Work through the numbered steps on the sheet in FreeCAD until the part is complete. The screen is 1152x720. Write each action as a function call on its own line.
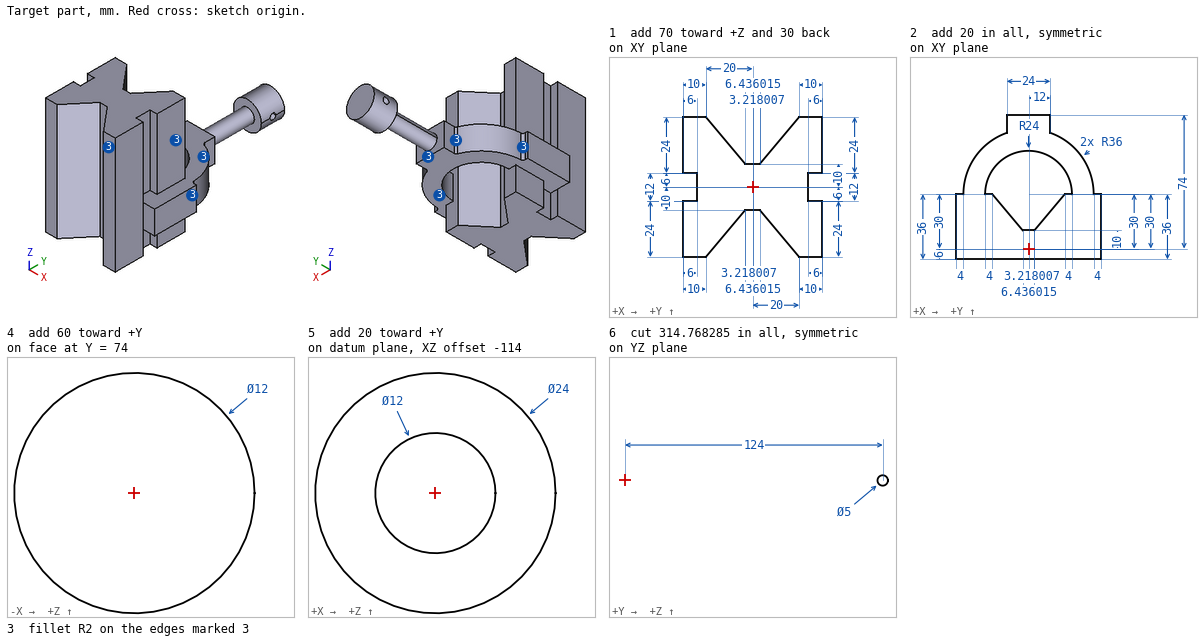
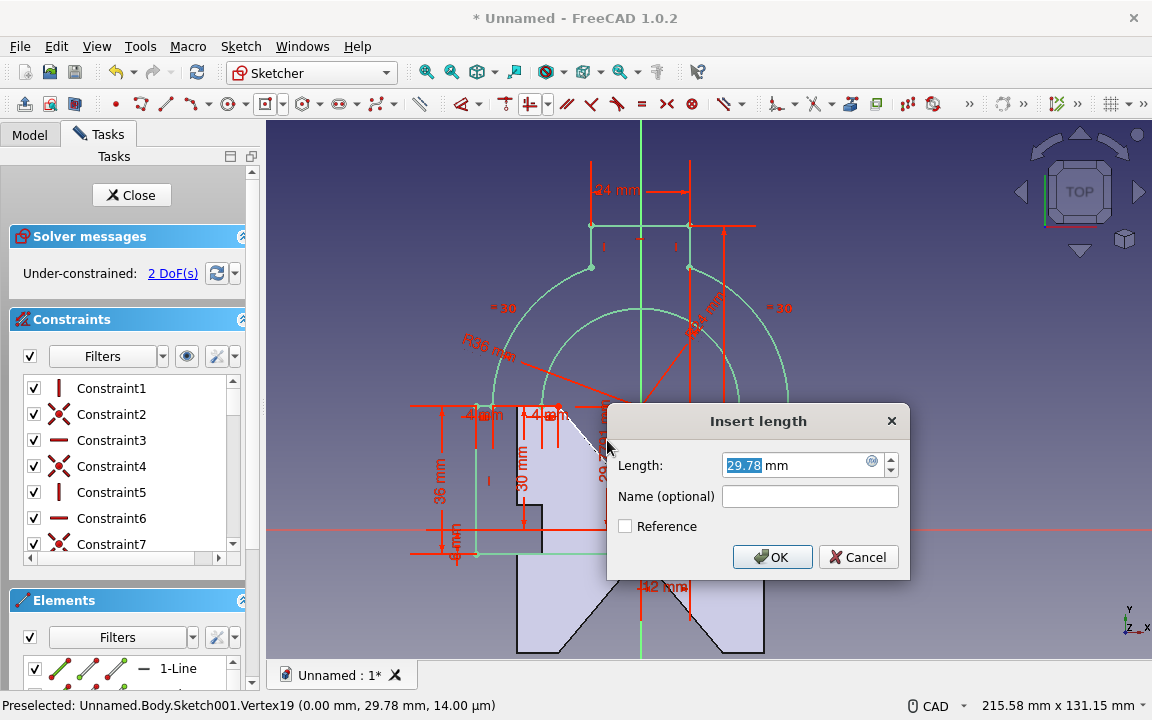
text(30)
key(Return)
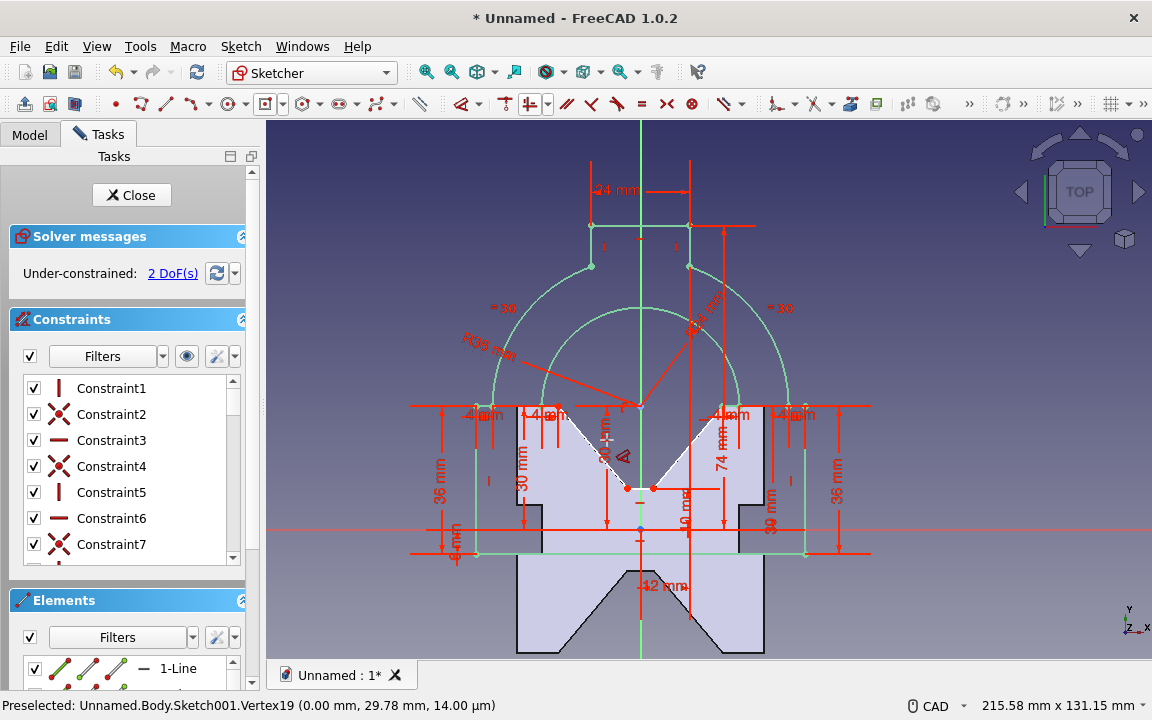
scroll(643, 489, up, 3)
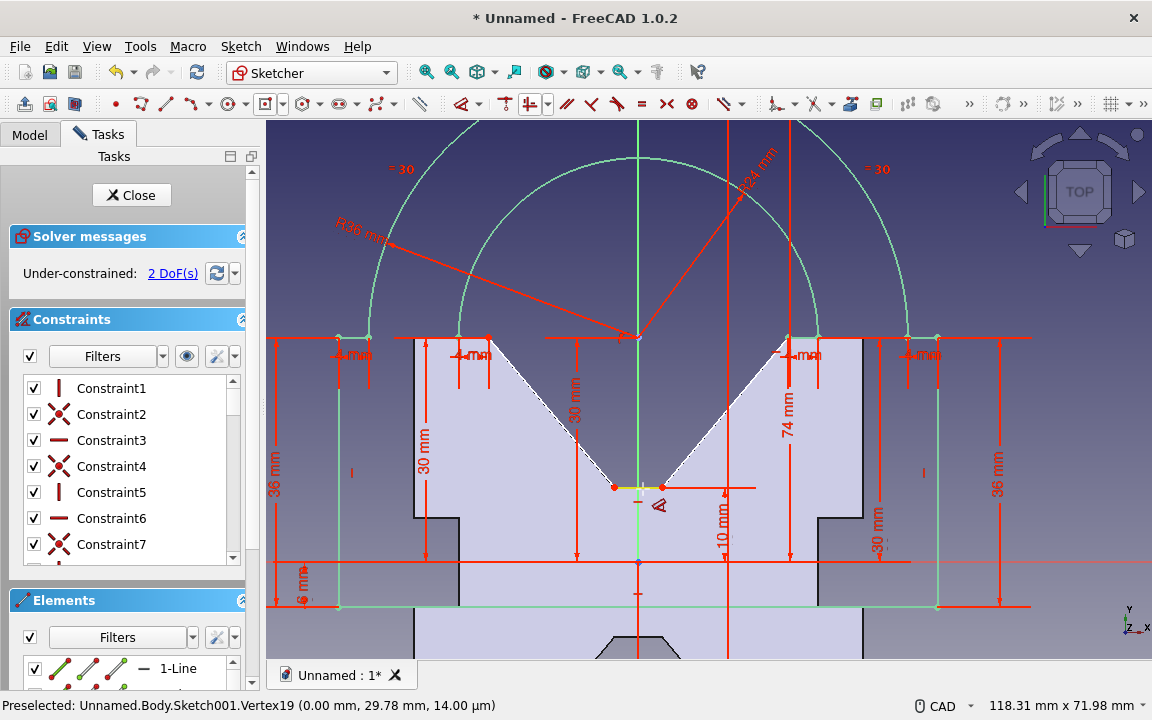
click(643, 488)
click(622, 522)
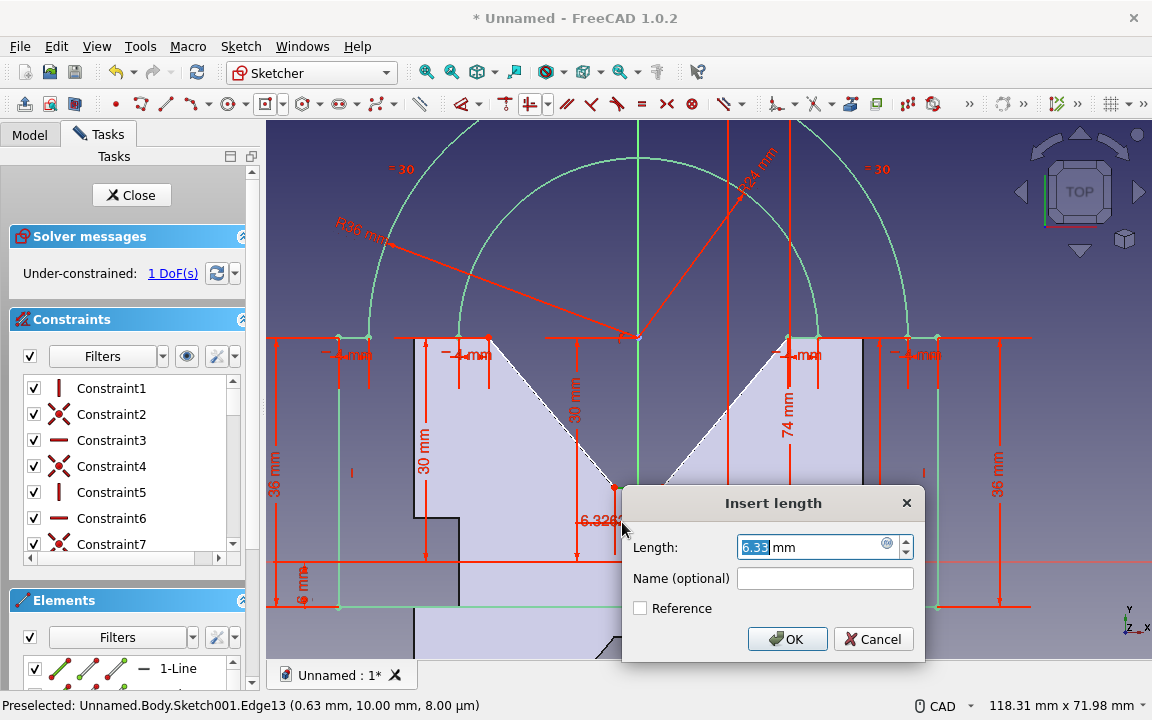
text(6.436015)
key(Return)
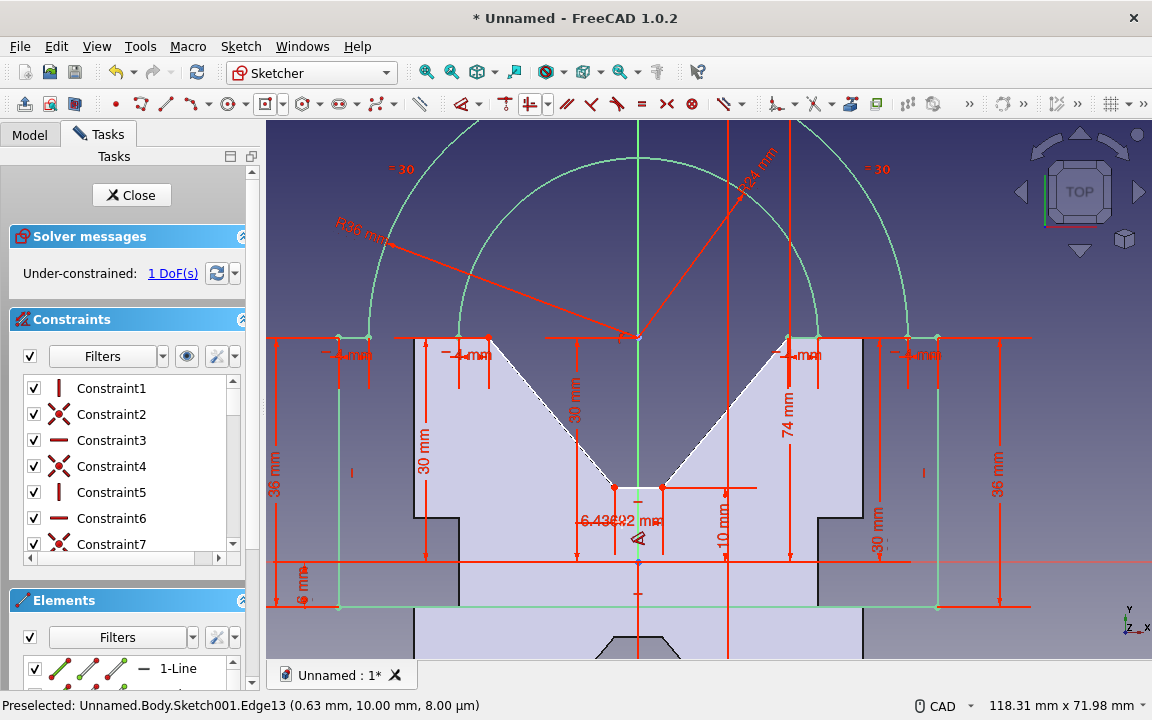
scroll(663, 488, up, 3)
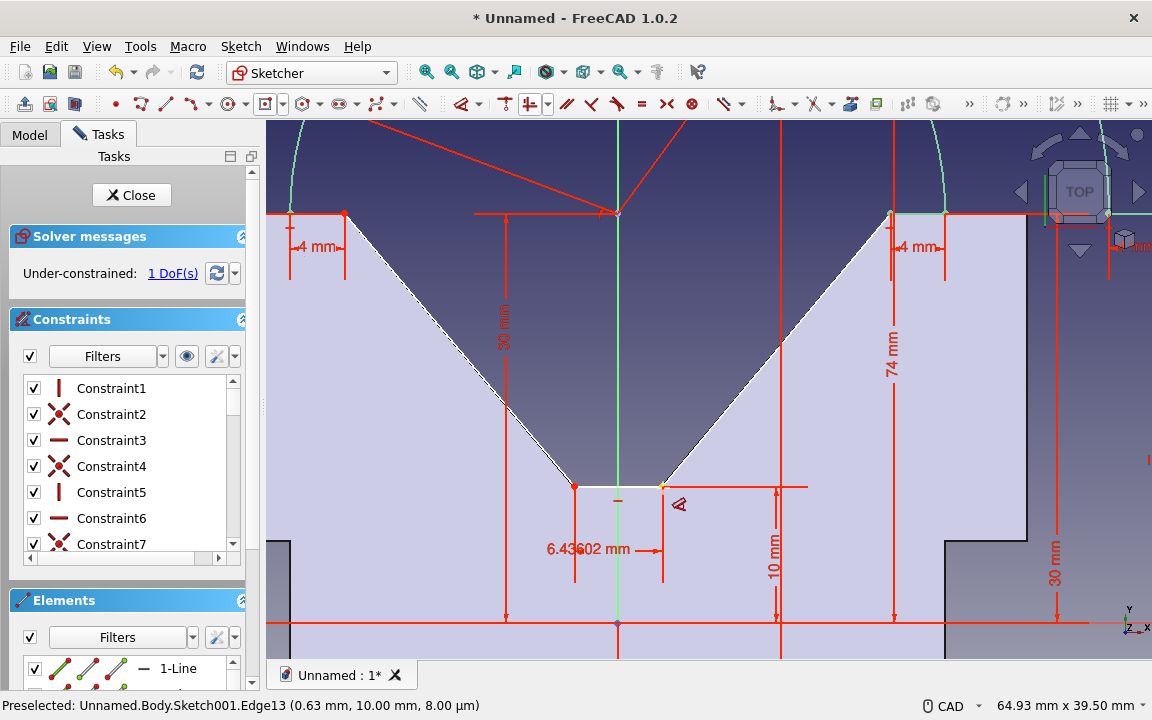
click(663, 487)
click(640, 453)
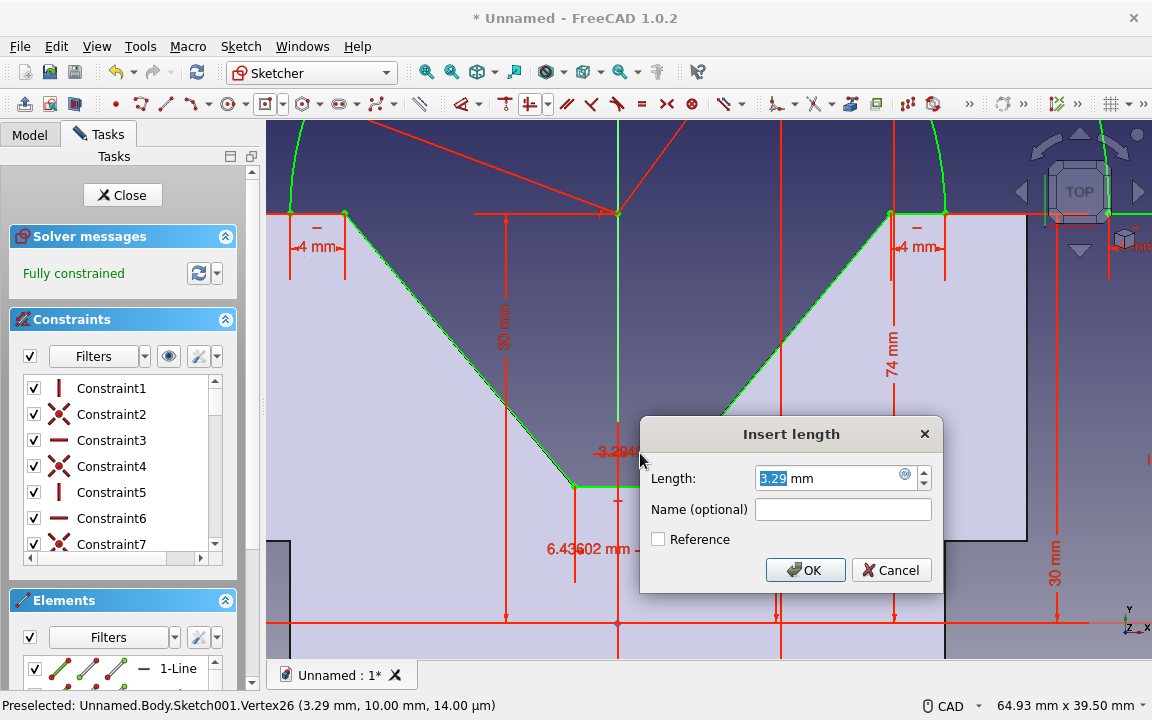
text(3.218007)
key(Return)
key(Escape)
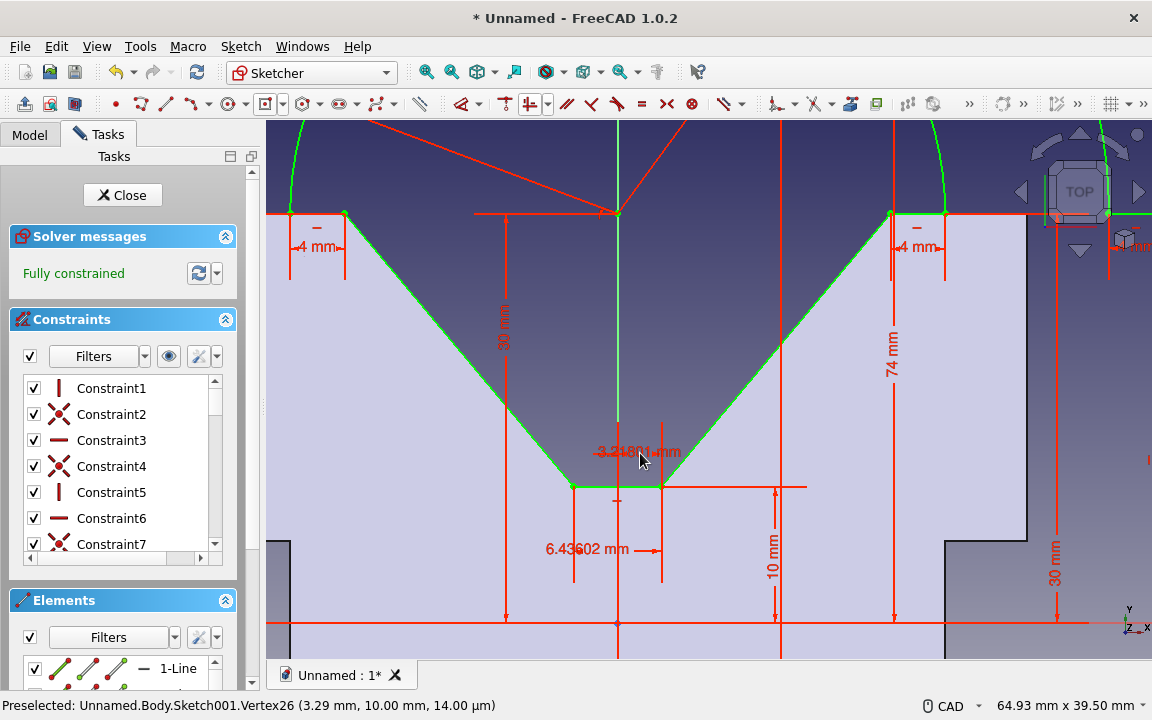
click(123, 195)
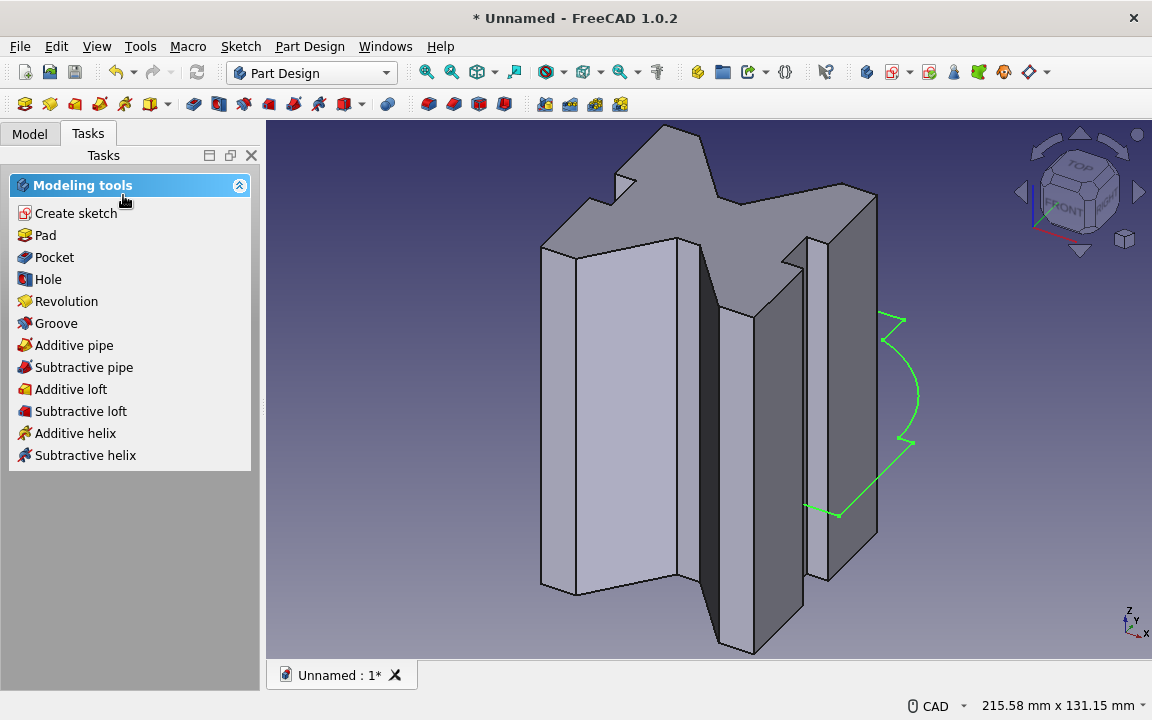
click(25, 104)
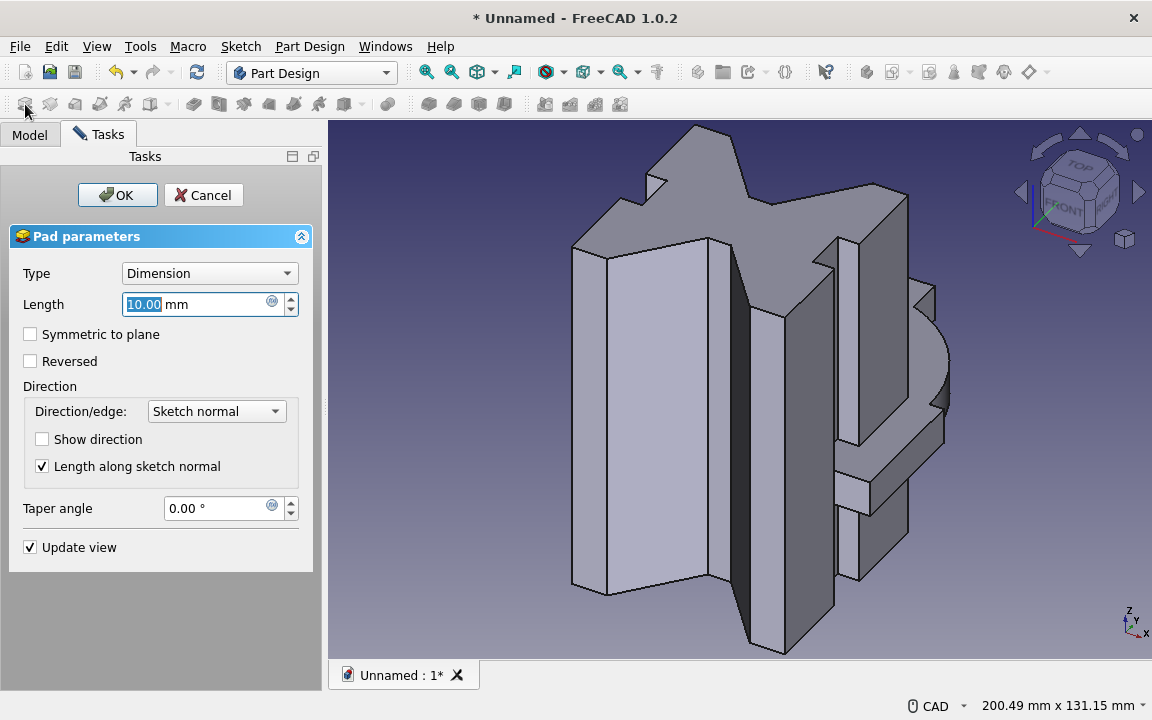
text(20)
key(Tab)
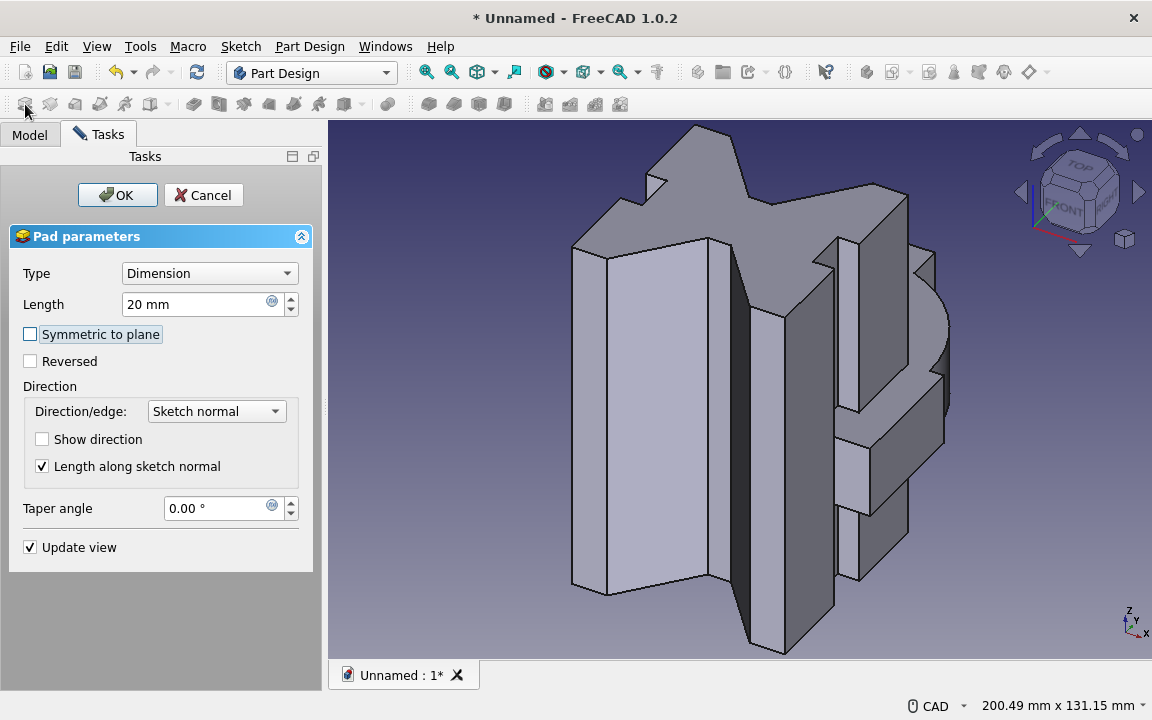
click(31, 334)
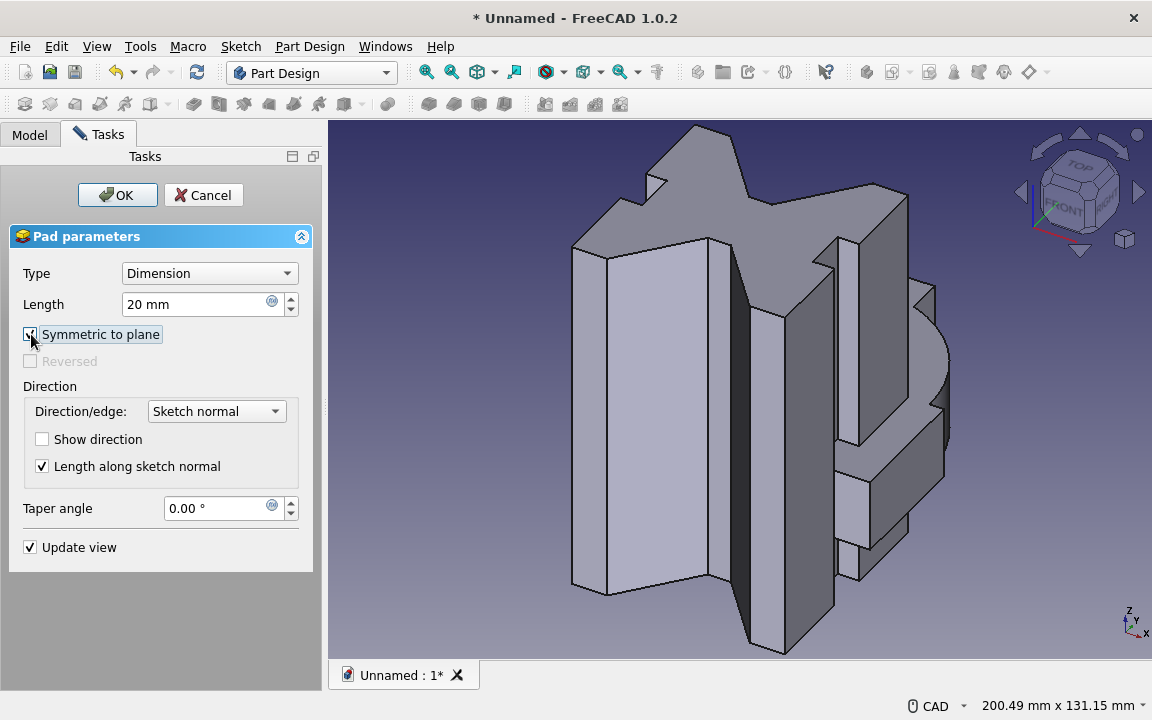
click(118, 195)